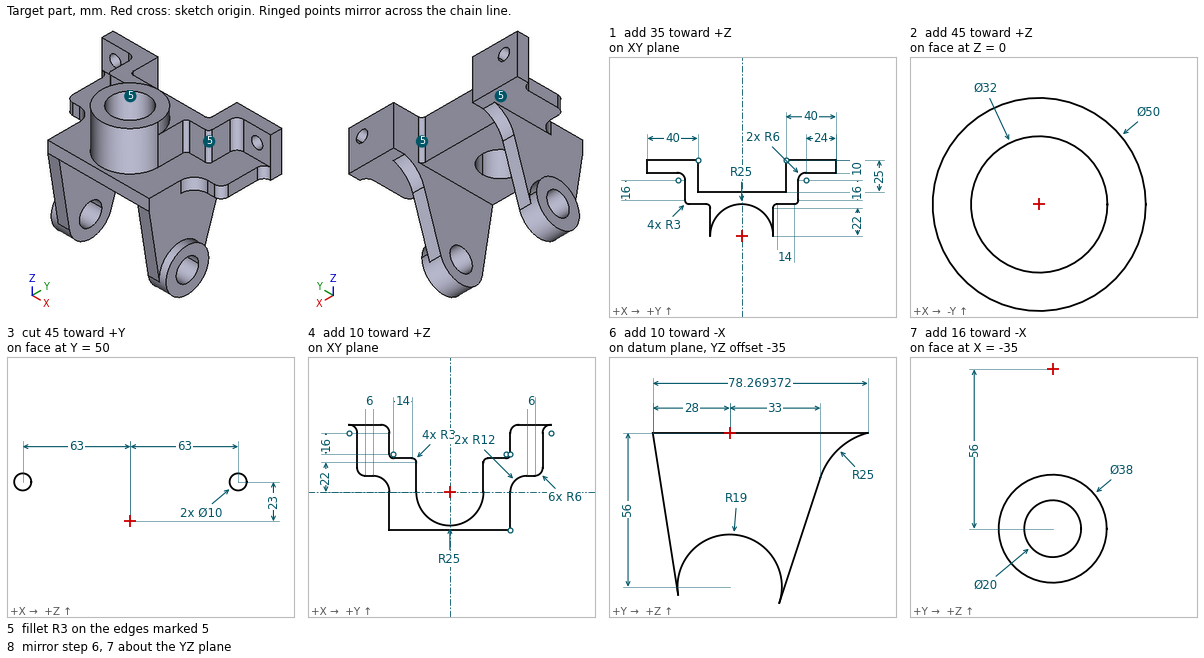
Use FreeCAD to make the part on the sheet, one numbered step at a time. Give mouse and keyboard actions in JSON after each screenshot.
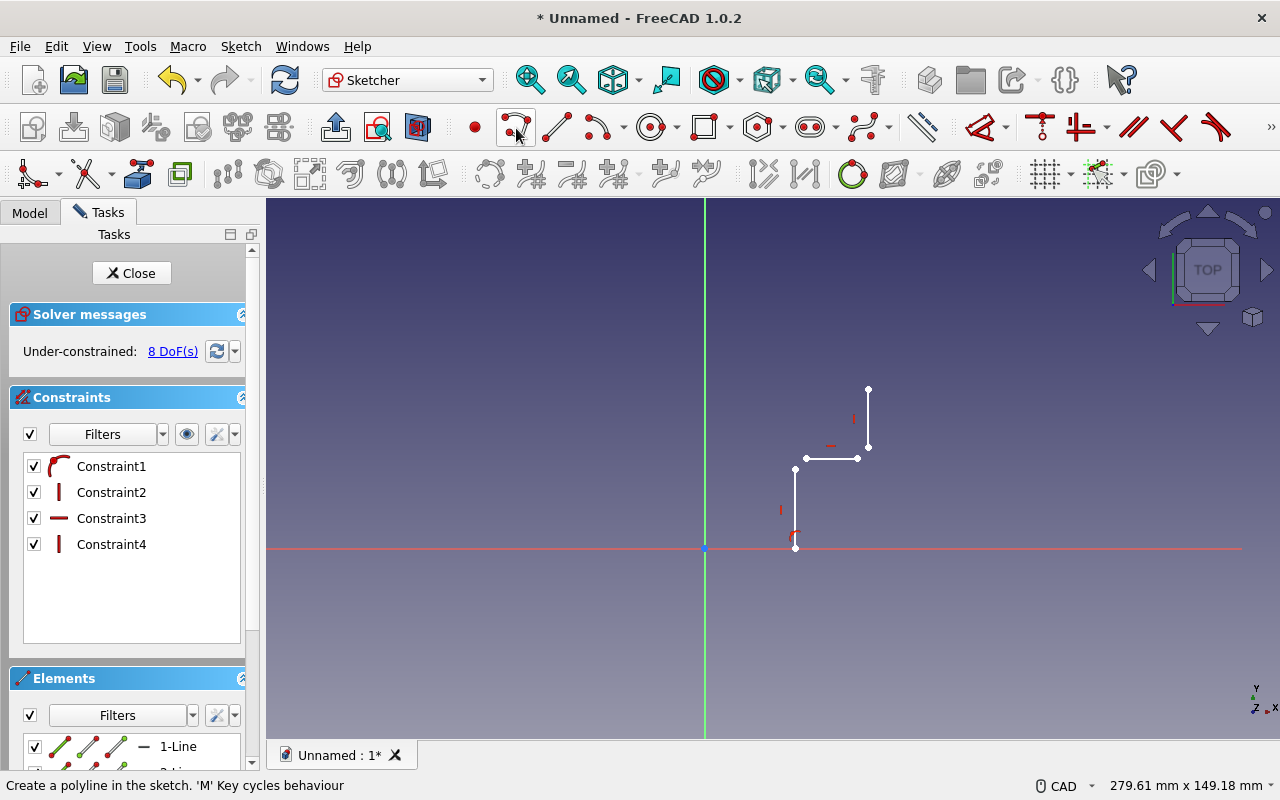
{"action": "left_click", "coordinate": [889, 367]}
{"action": "left_click", "coordinate": [977, 367]}
{"action": "left_click", "coordinate": [977, 331]}
{"action": "left_click", "coordinate": [831, 331]}
{"action": "left_click", "coordinate": [831, 422]}
{"action": "left_click", "coordinate": [578, 422]}
{"action": "left_click", "coordinate": [578, 331]}
{"action": "left_click", "coordinate": [433, 331]}
{"action": "left_click", "coordinate": [433, 367]}
{"action": "left_click", "coordinate": [520, 367]}
{"action": "right_click", "coordinate": [520, 367]}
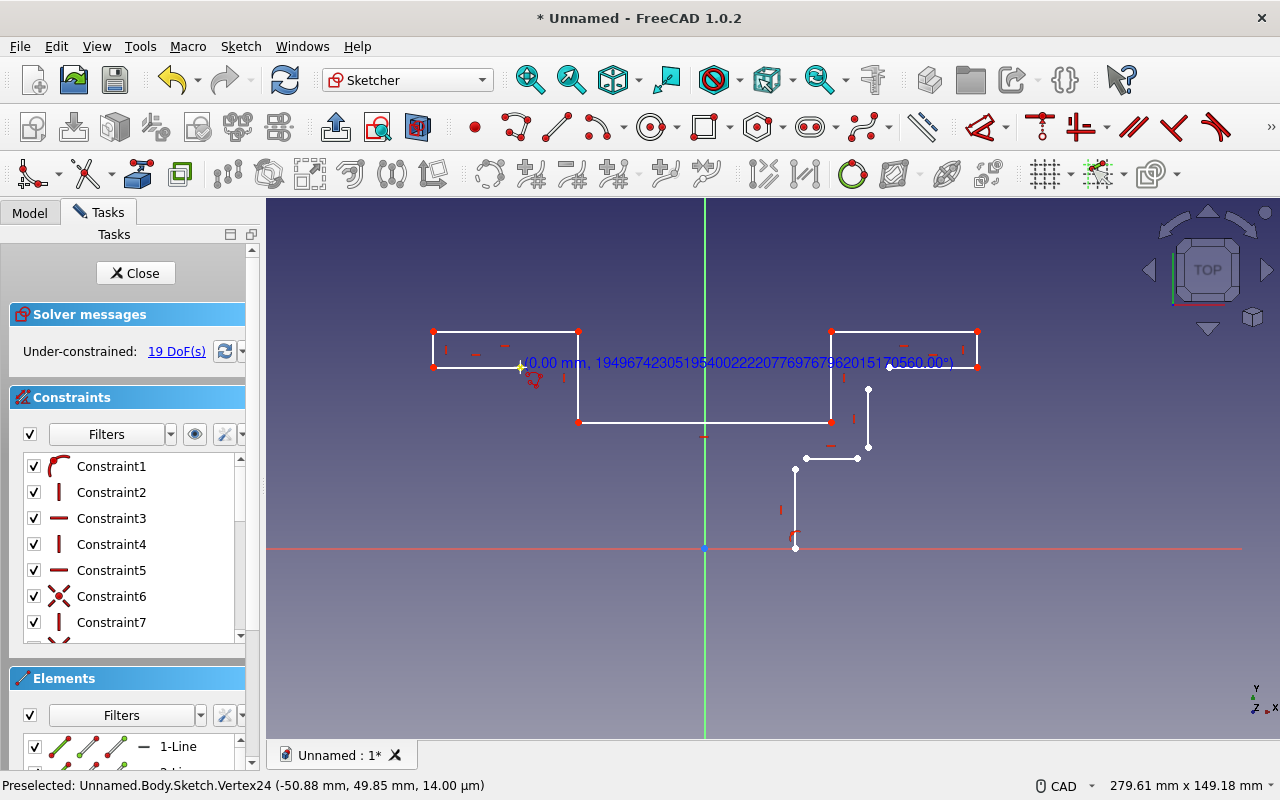
{"action": "left_click", "coordinate": [557, 128]}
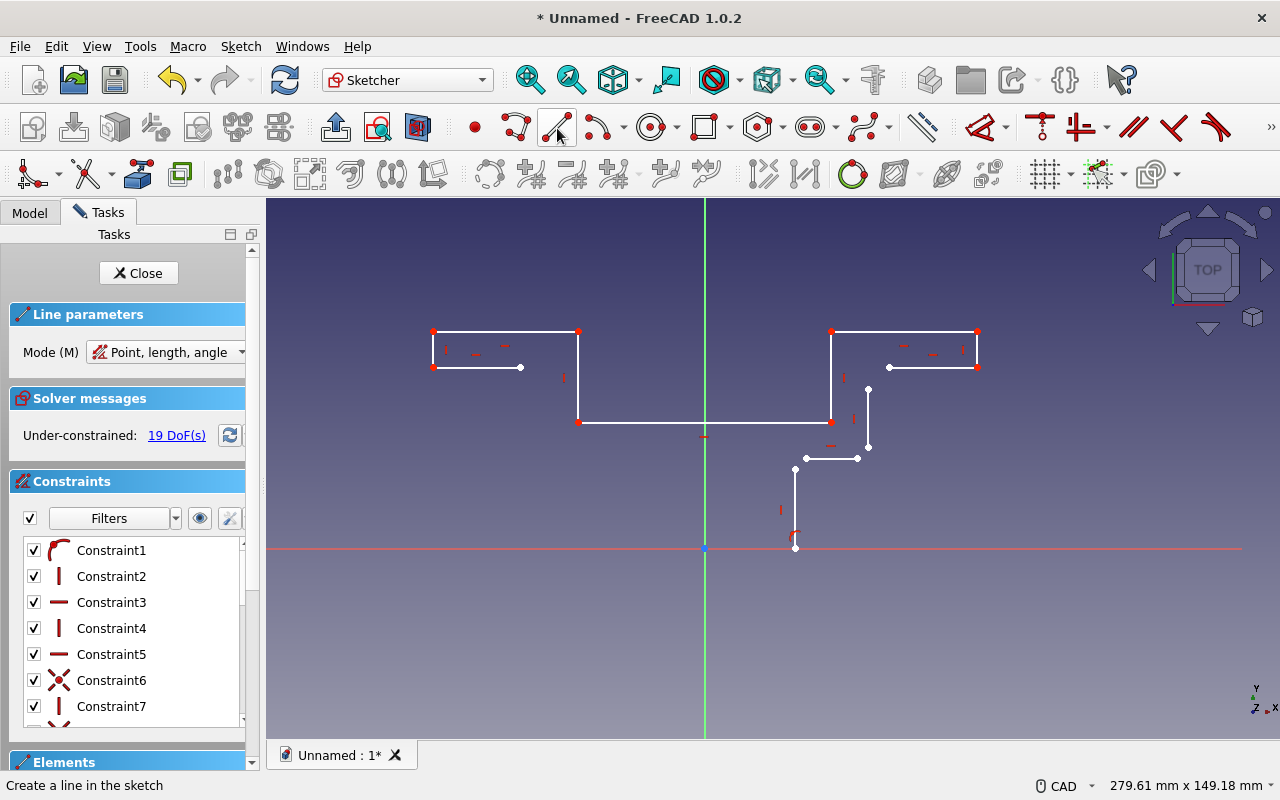
{"action": "left_click", "coordinate": [541, 389]}
{"action": "left_click", "coordinate": [541, 447]}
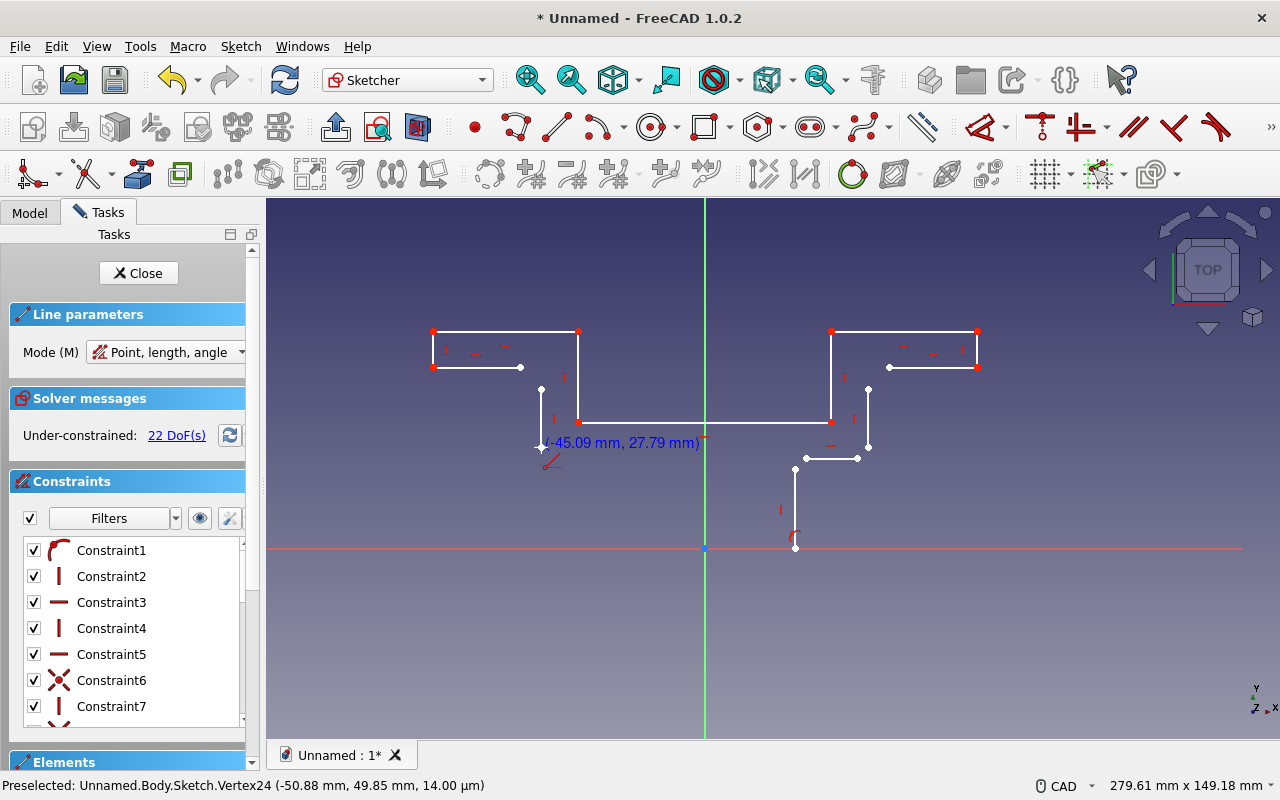
{"action": "left_click", "coordinate": [552, 458]}
{"action": "left_click", "coordinate": [603, 458]}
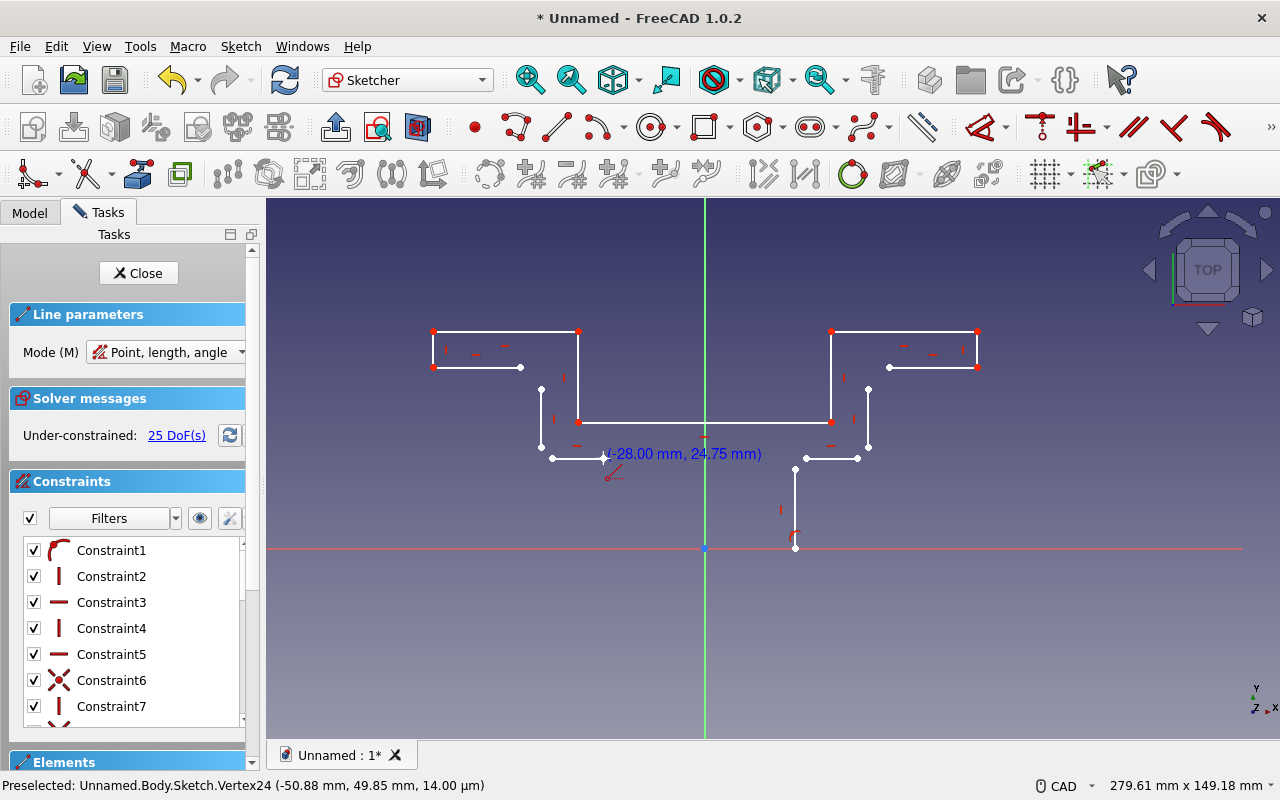
{"action": "left_click", "coordinate": [614, 469]}
{"action": "left_click", "coordinate": [614, 549]}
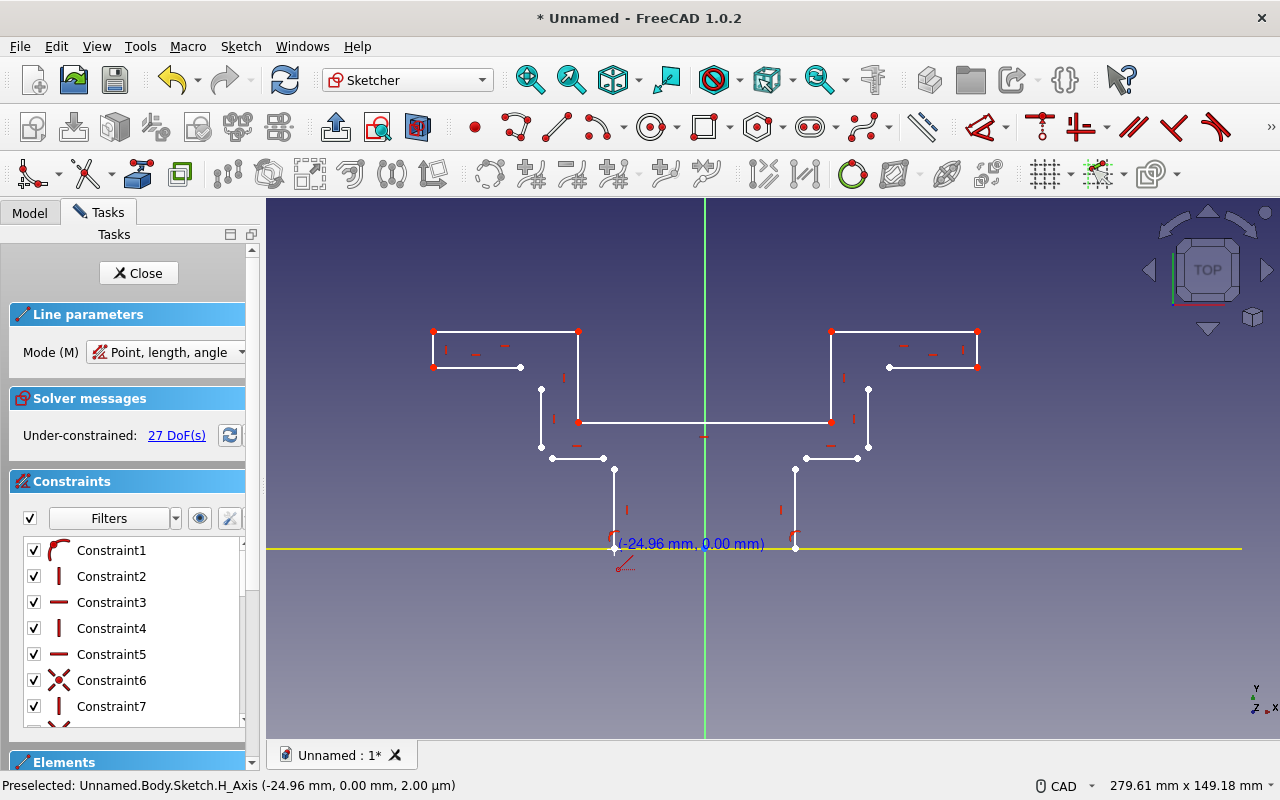
{"action": "left_click", "coordinate": [624, 128]}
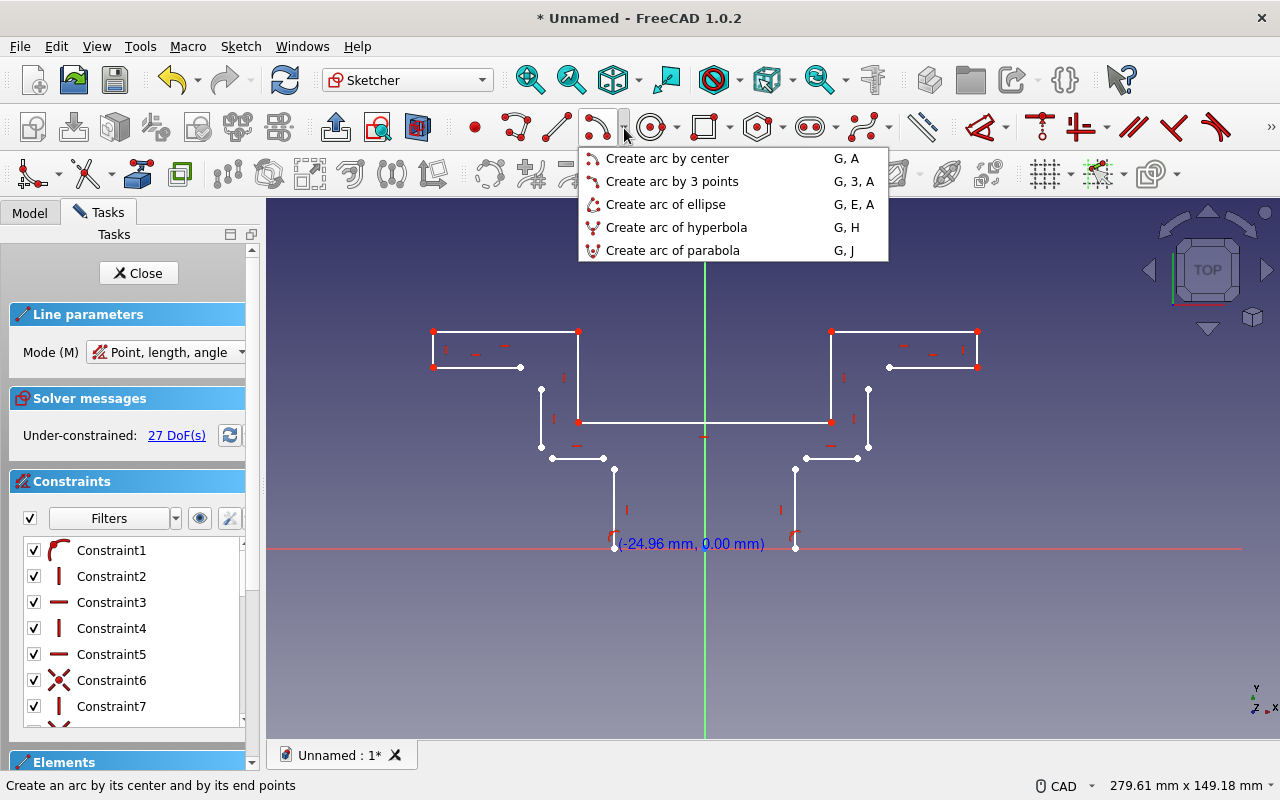
{"action": "left_click", "coordinate": [734, 182]}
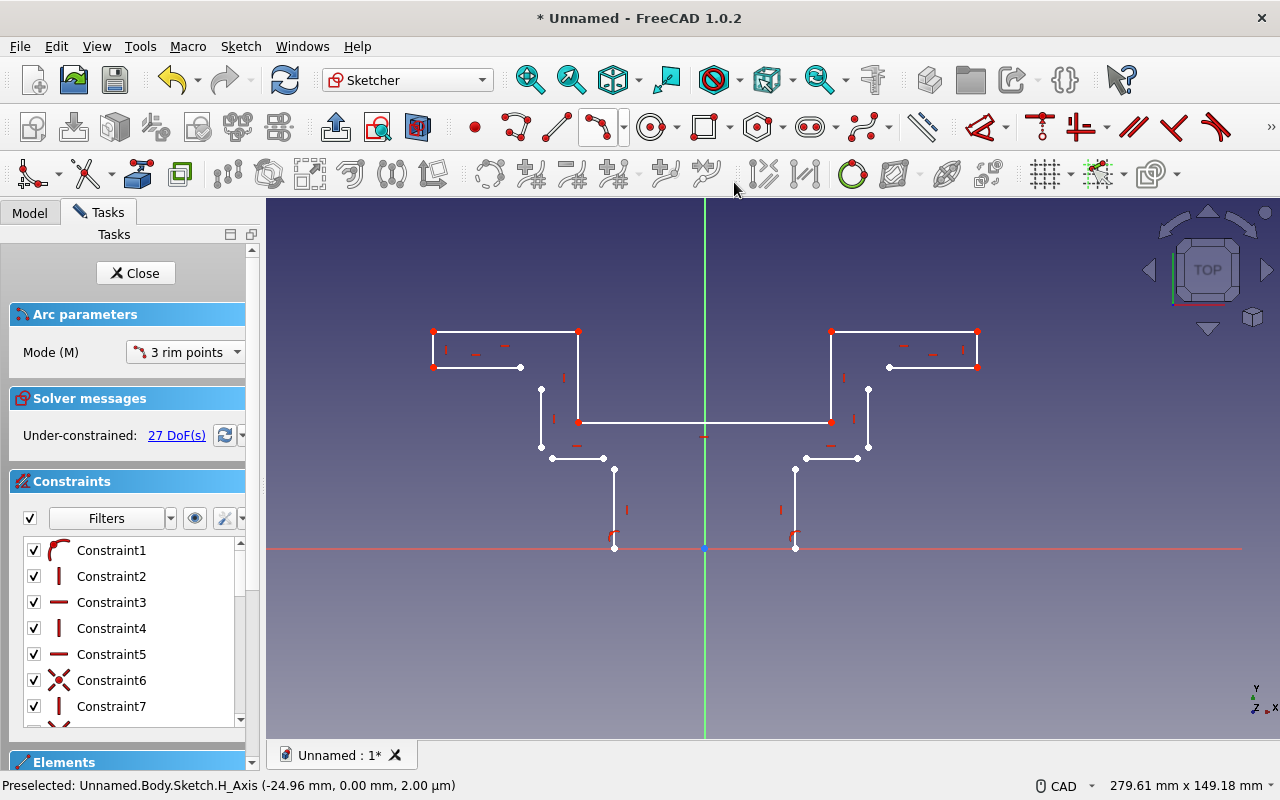
{"action": "left_click", "coordinate": [795, 470]}
{"action": "left_click", "coordinate": [806, 459]}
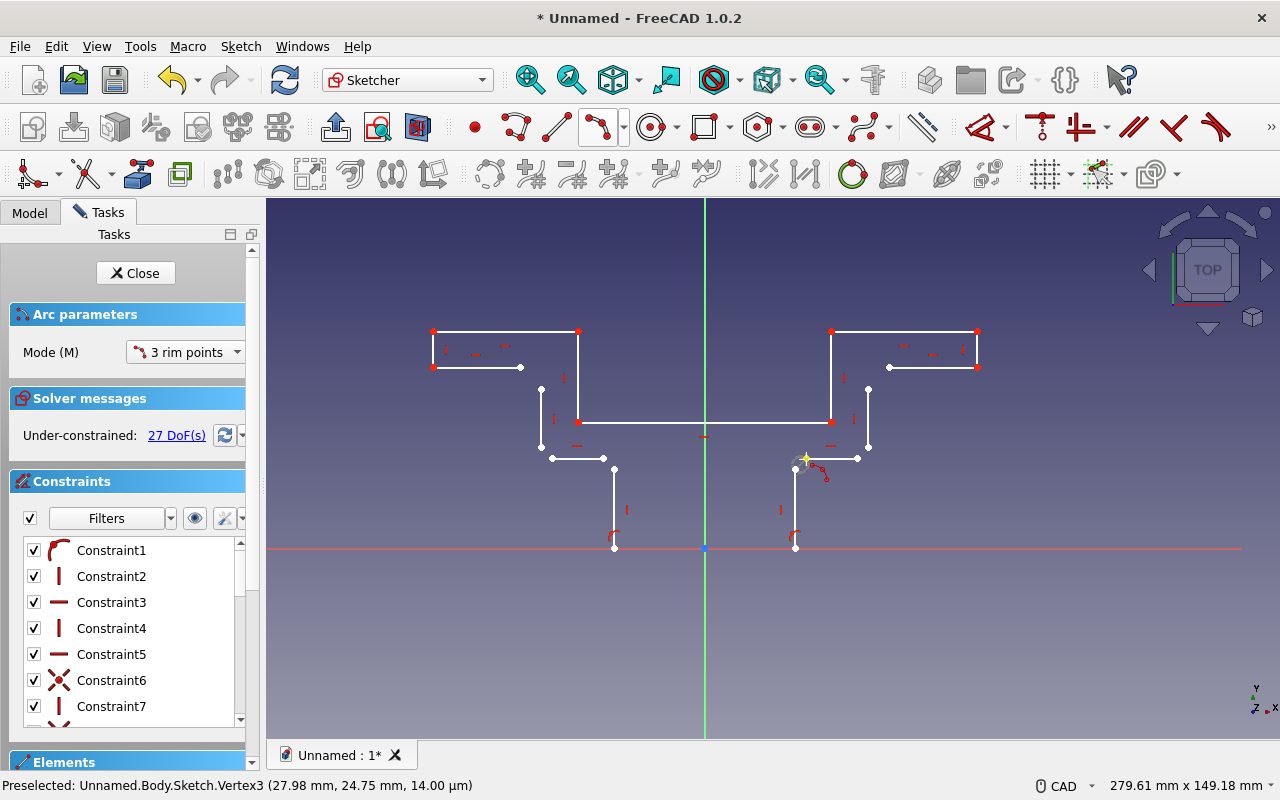
{"action": "scroll", "coordinate": [798, 461], "scroll_direction": "up", "scroll_amount": 9}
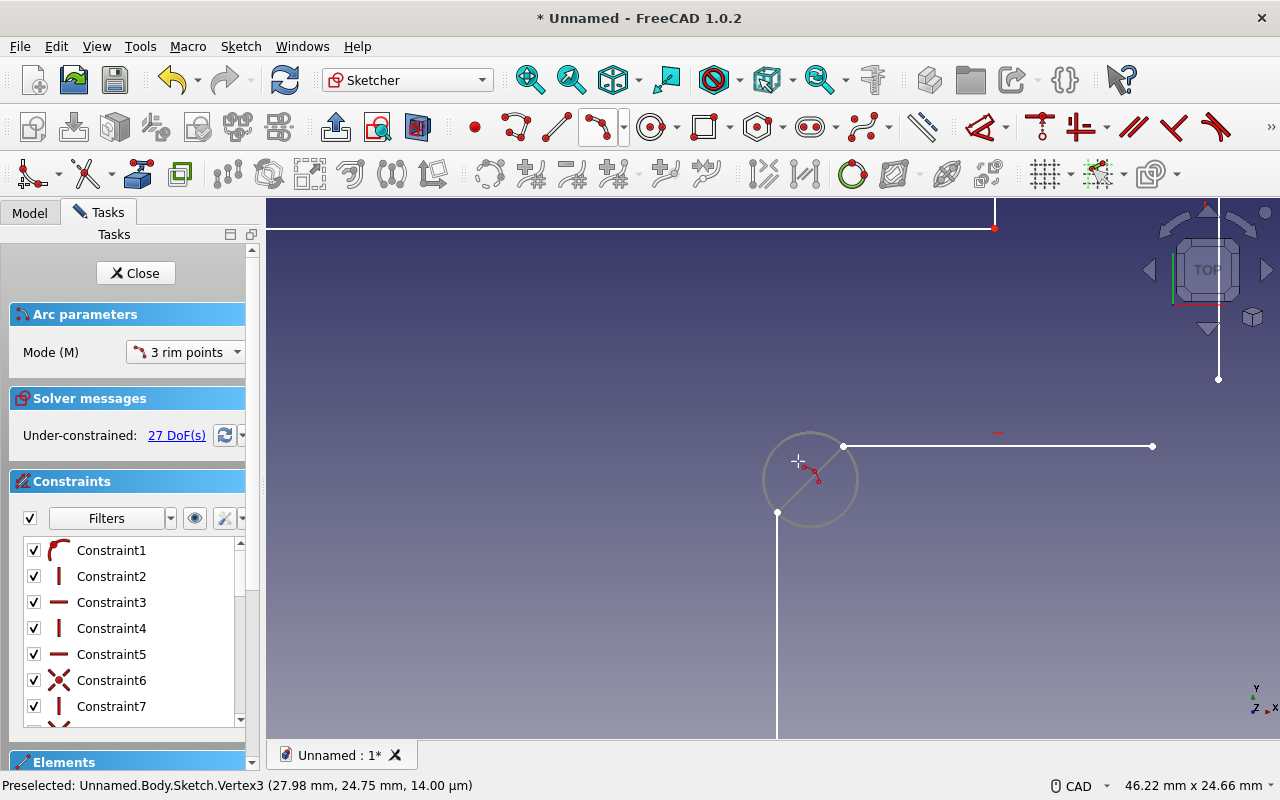
{"action": "left_click", "coordinate": [798, 460]}